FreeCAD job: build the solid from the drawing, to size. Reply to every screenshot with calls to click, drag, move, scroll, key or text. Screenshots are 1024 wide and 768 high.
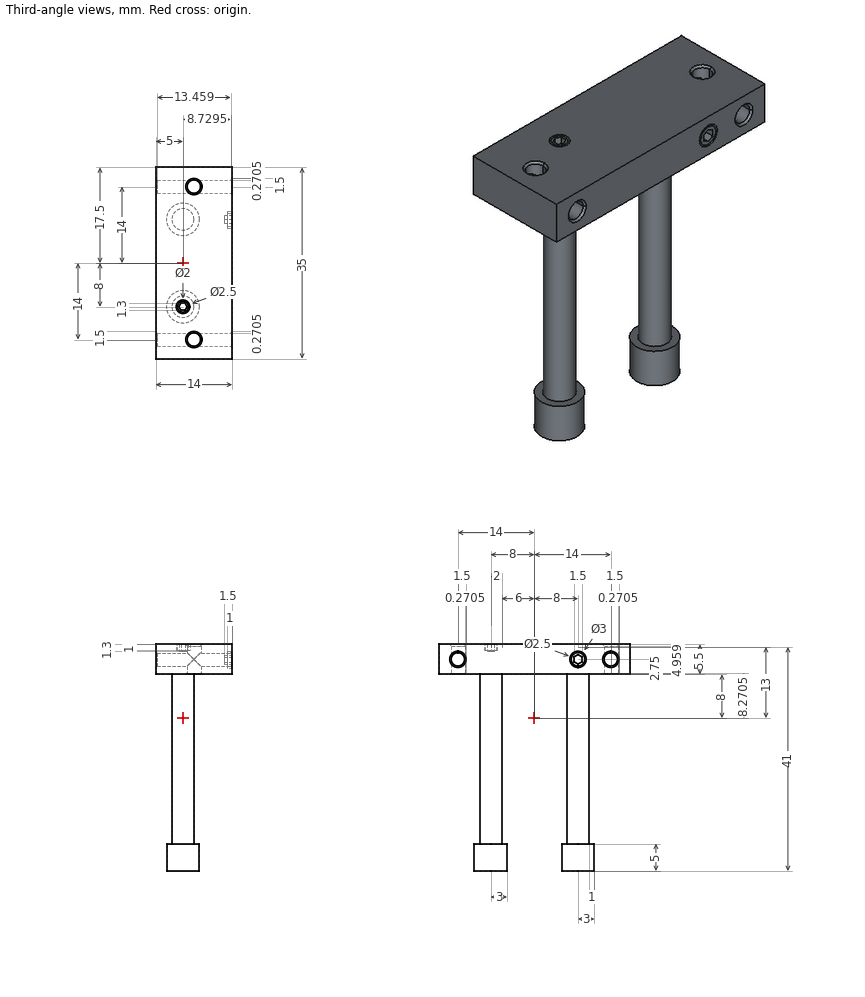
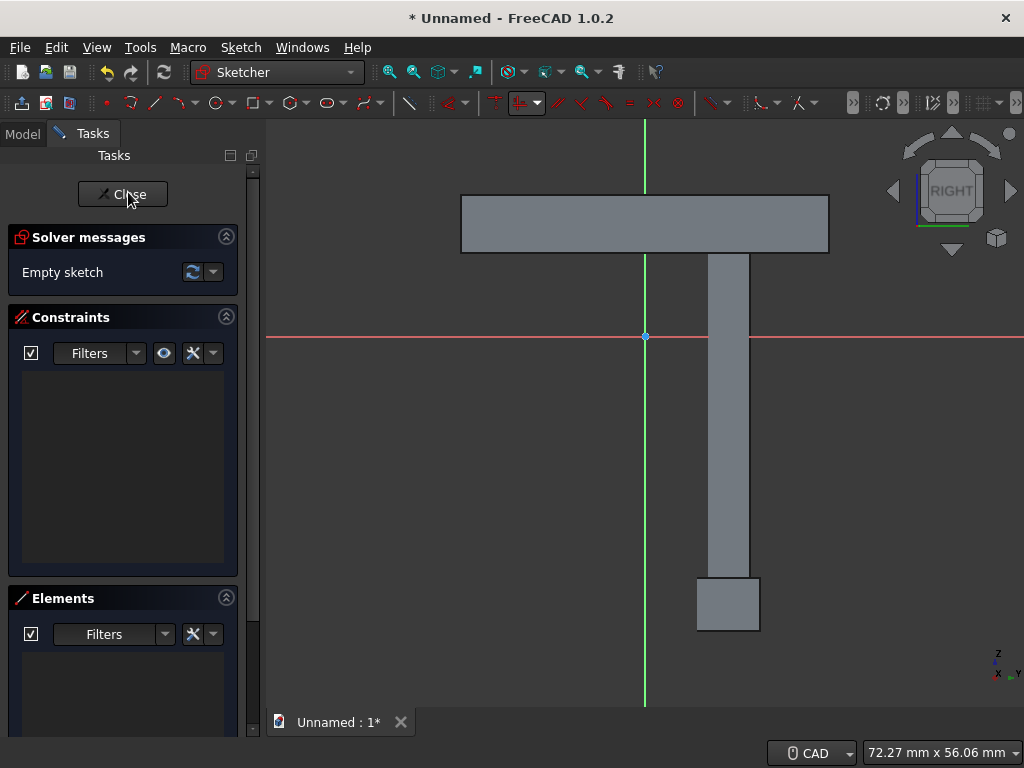
click(70, 104)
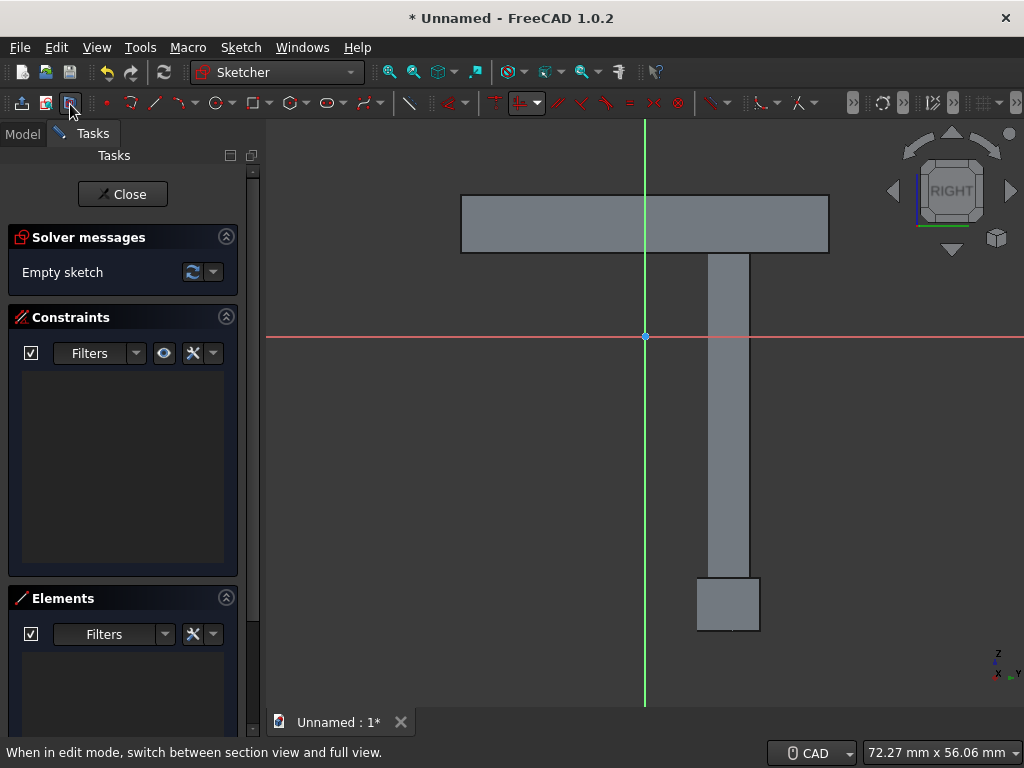
scroll(523, 583, down, 2)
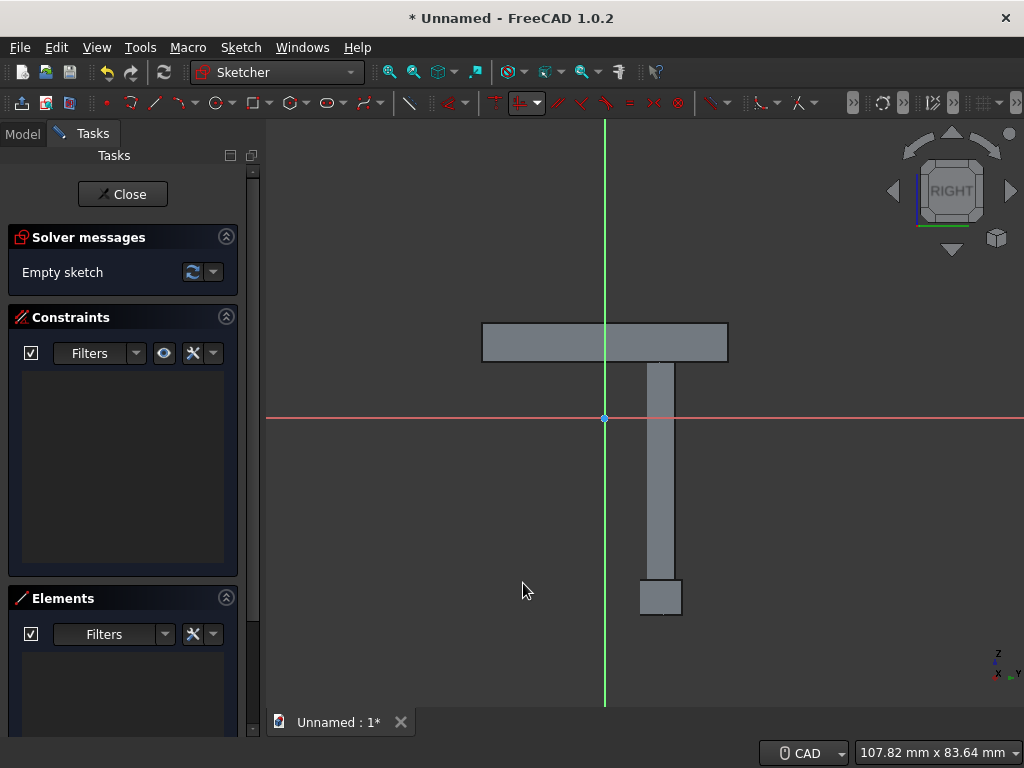
click(132, 104)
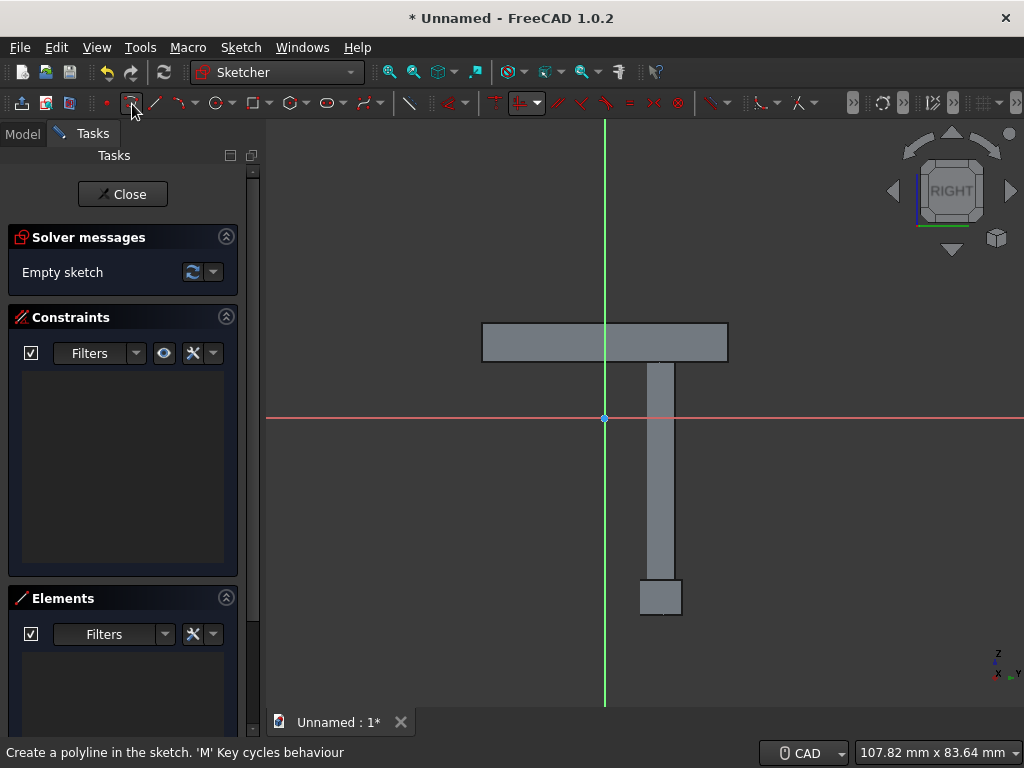
click(563, 327)
click(549, 327)
click(549, 615)
click(570, 615)
click(570, 580)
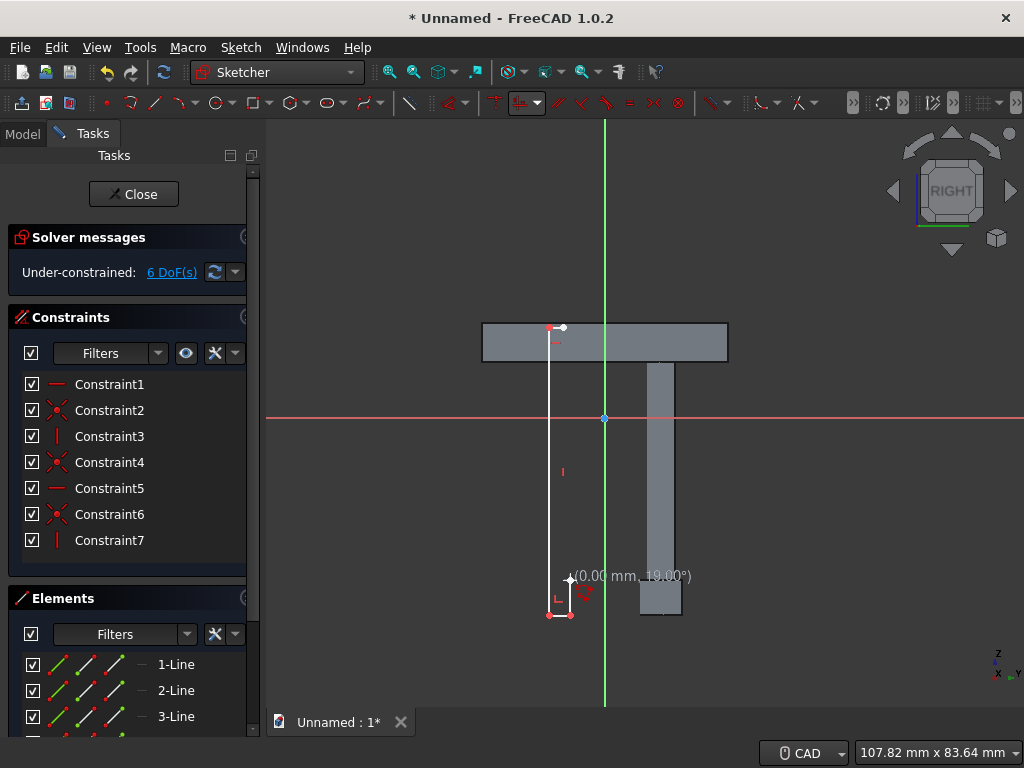
scroll(563, 580, up, 5)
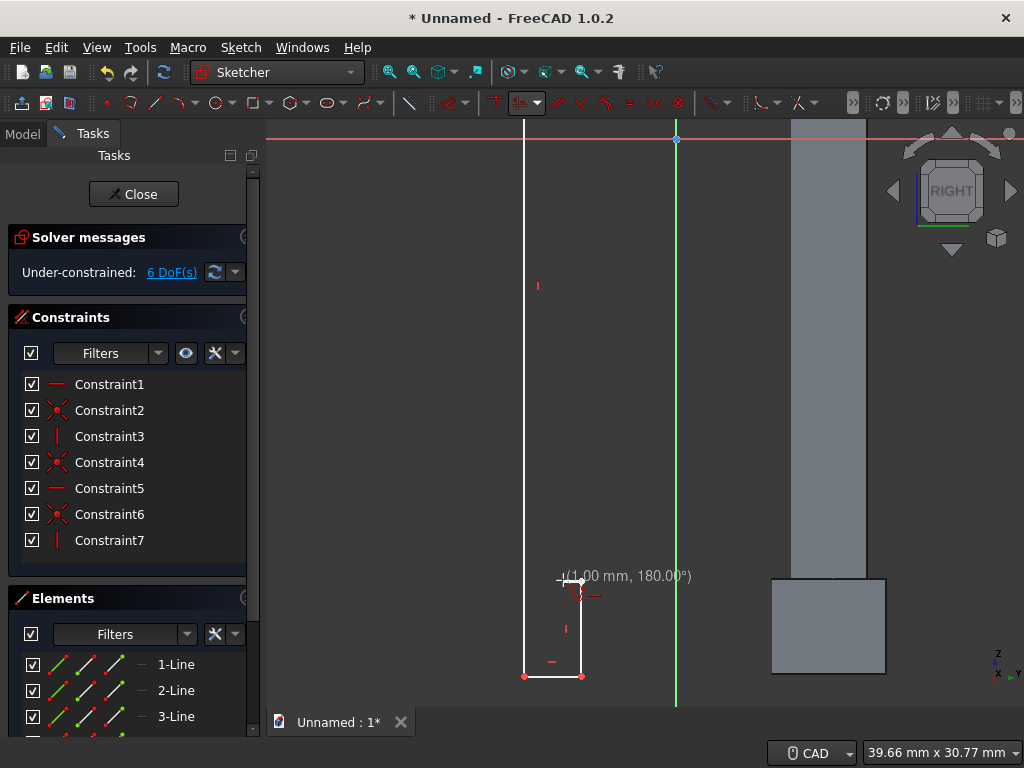
click(562, 579)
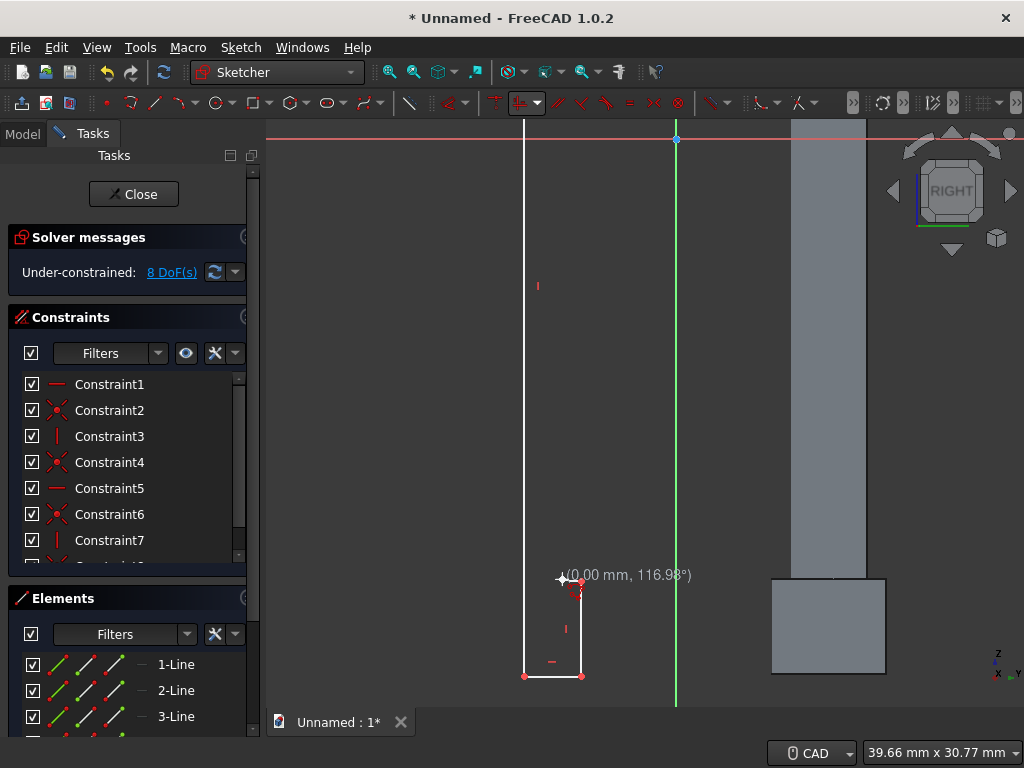
scroll(563, 580, down, 5)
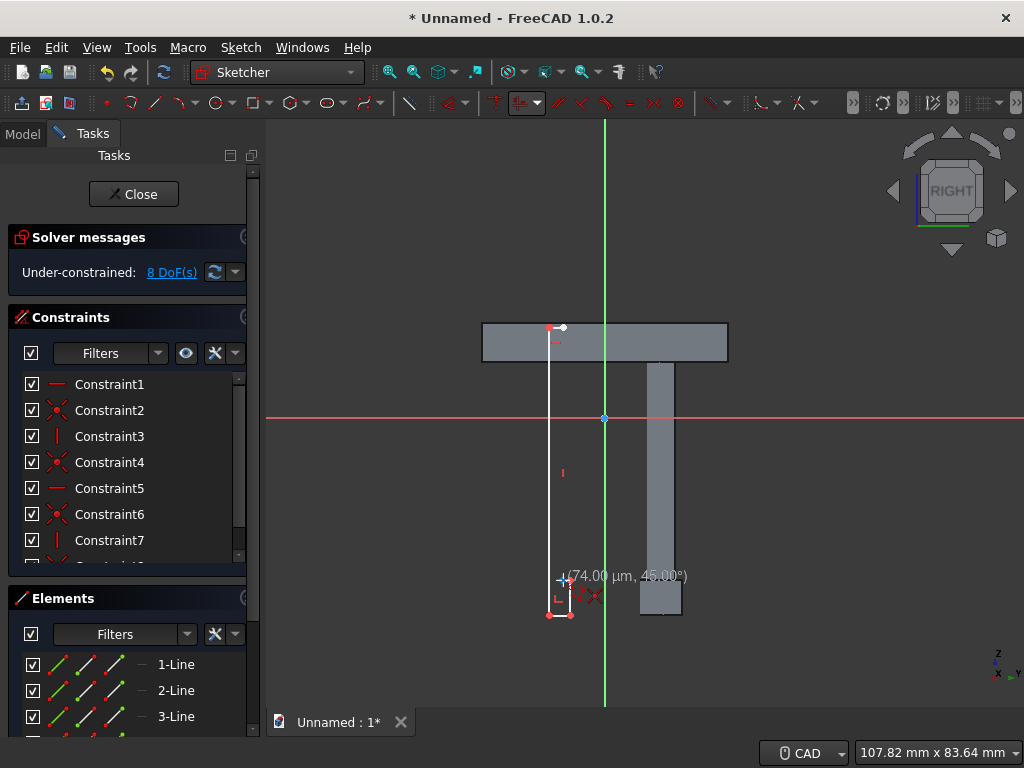
scroll(563, 327, up, 5)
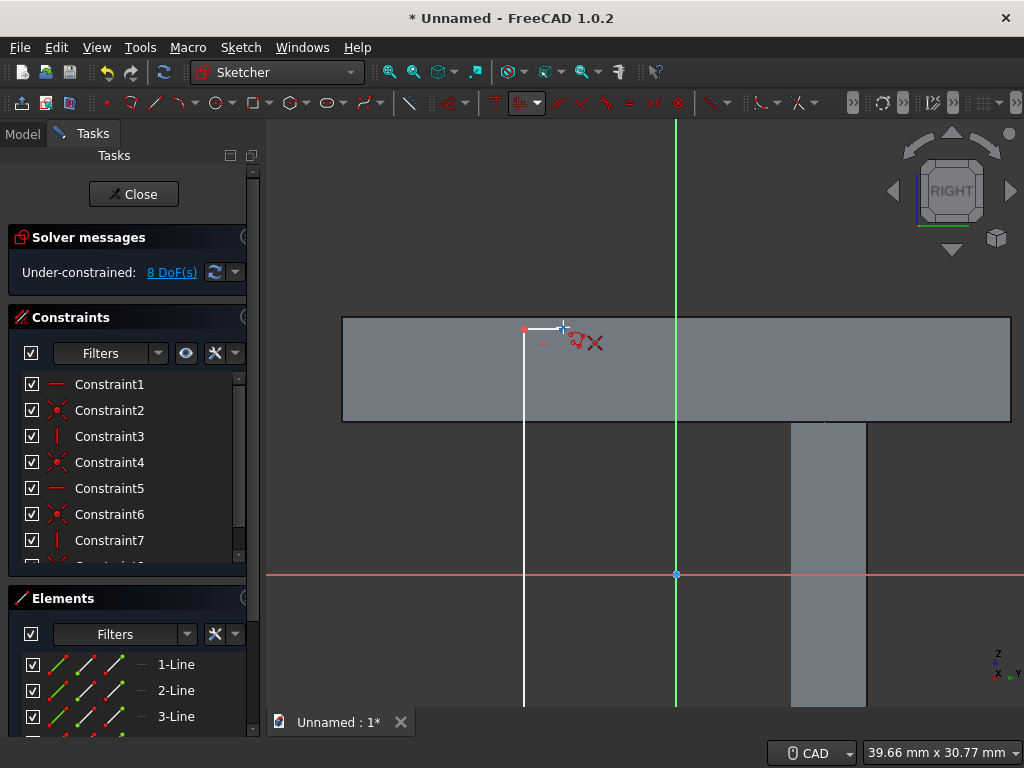
click(562, 329)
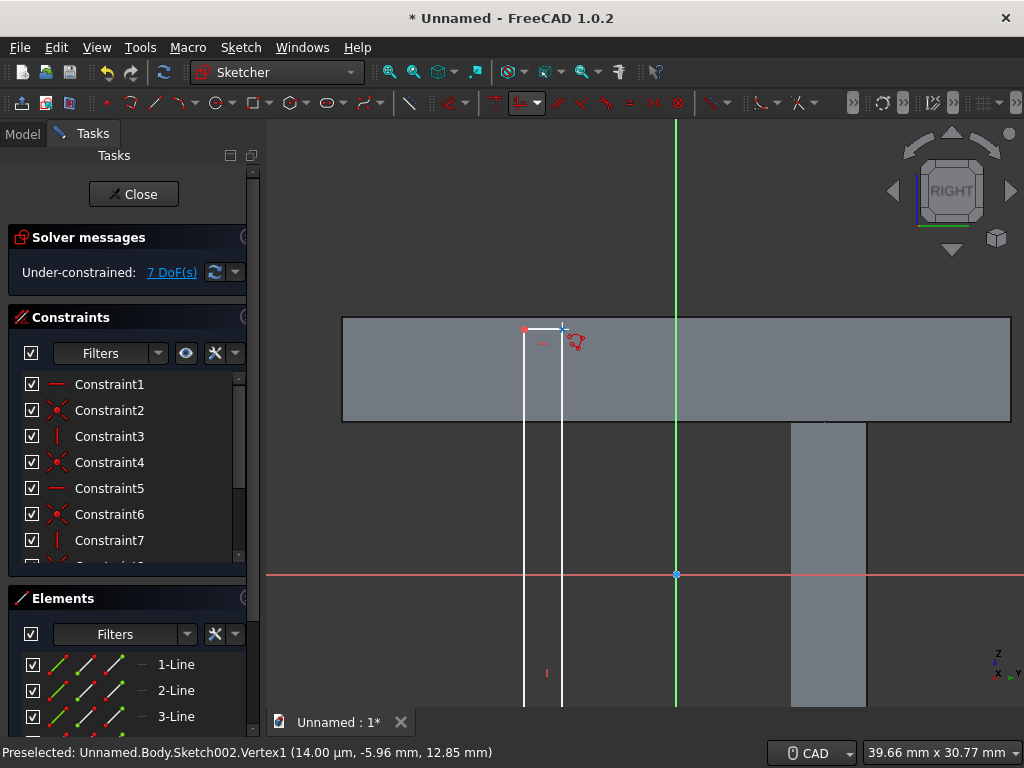
click(156, 104)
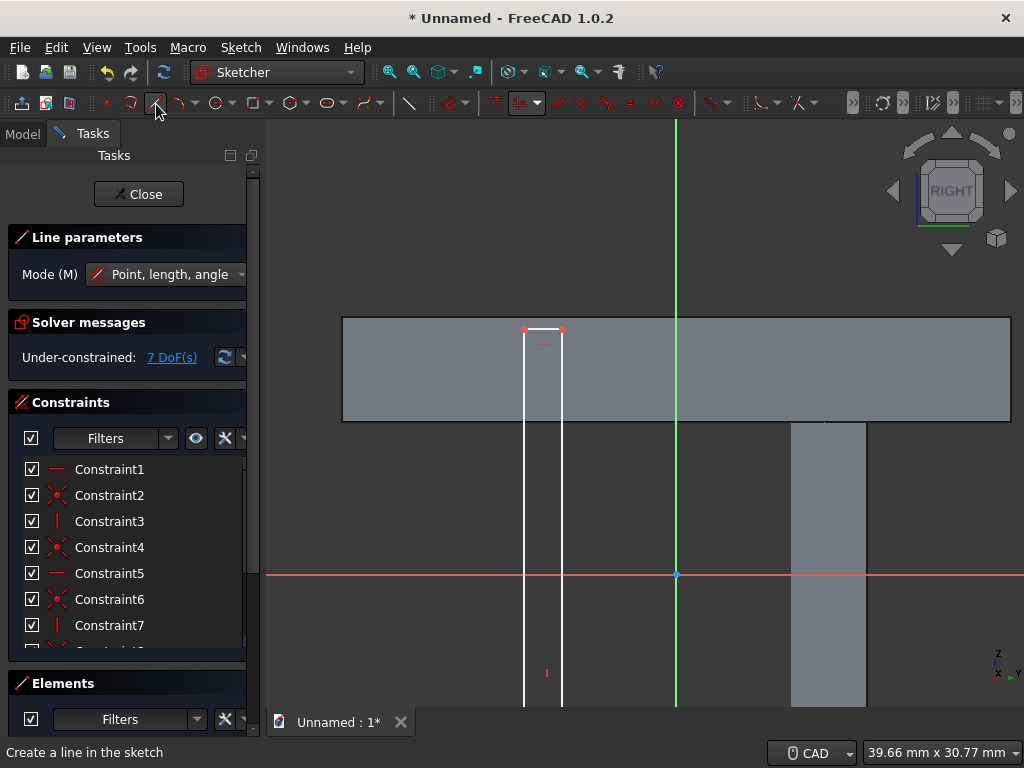
click(523, 248)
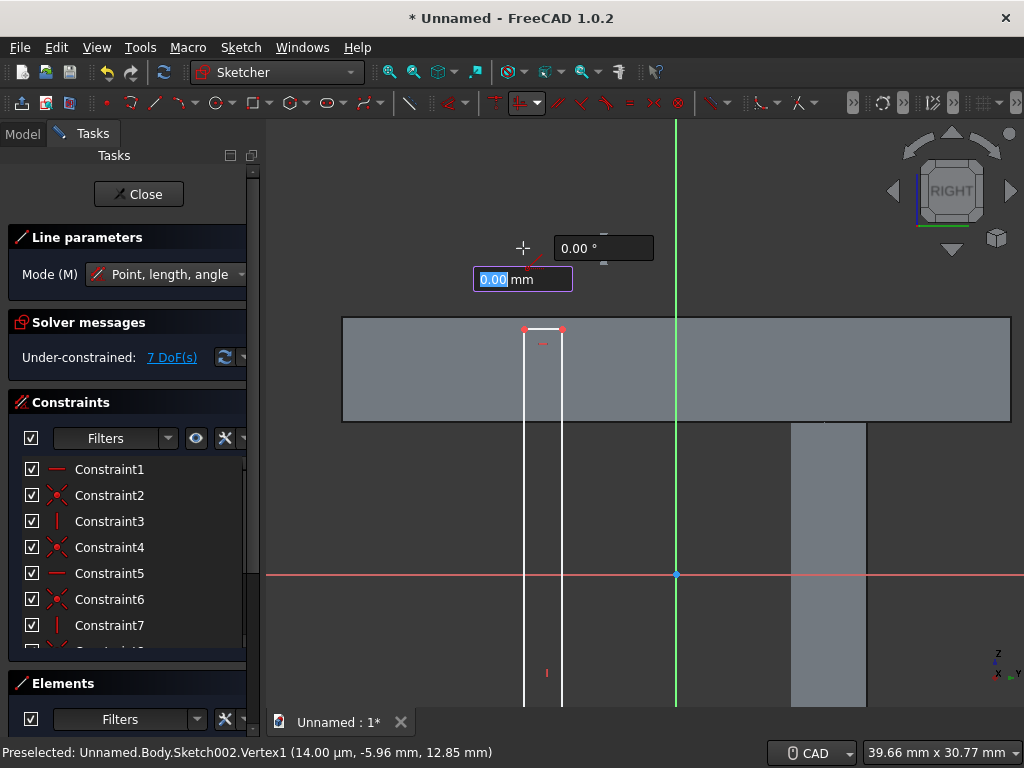
scroll(563, 327, down, 5)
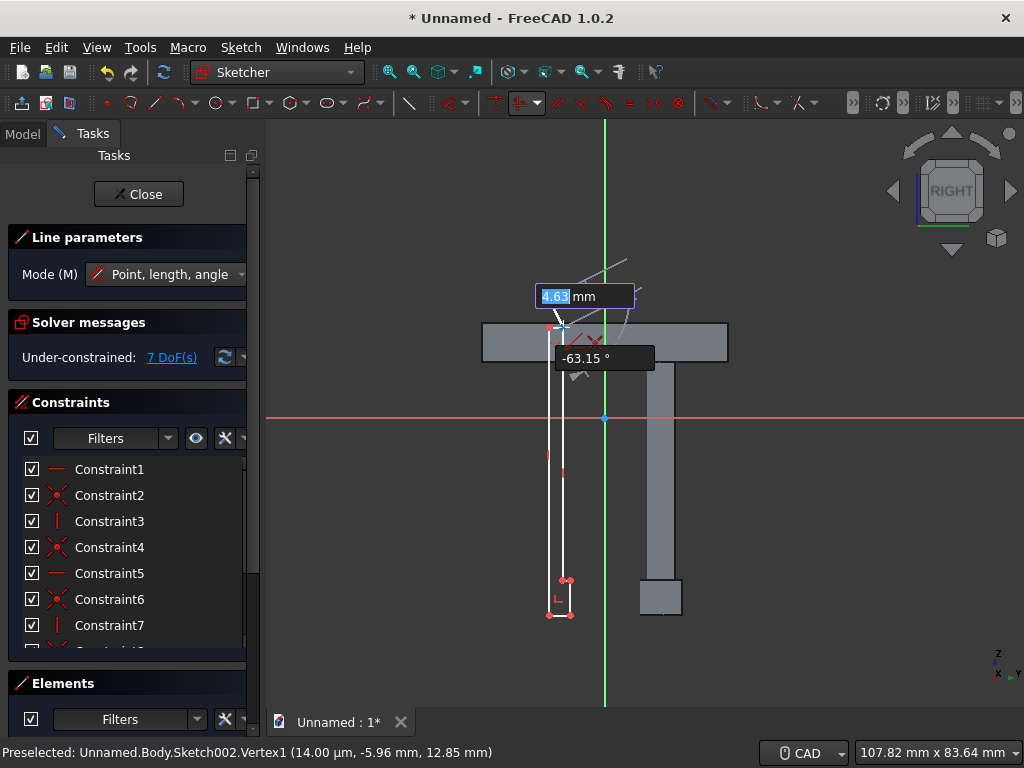
click(549, 212)
key(Escape)